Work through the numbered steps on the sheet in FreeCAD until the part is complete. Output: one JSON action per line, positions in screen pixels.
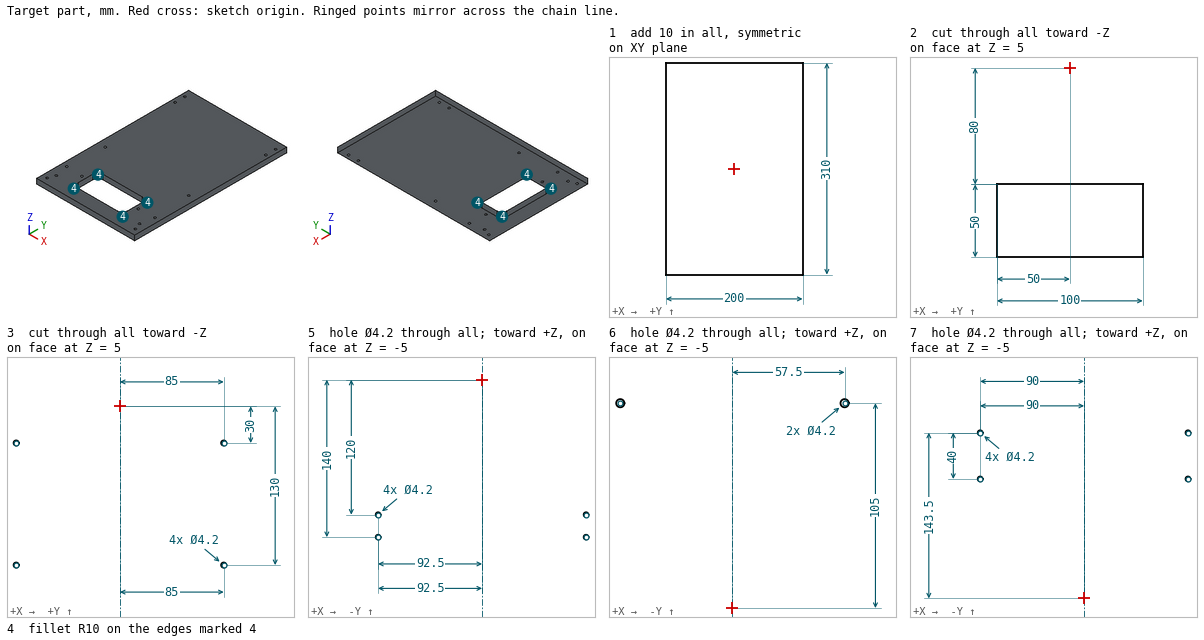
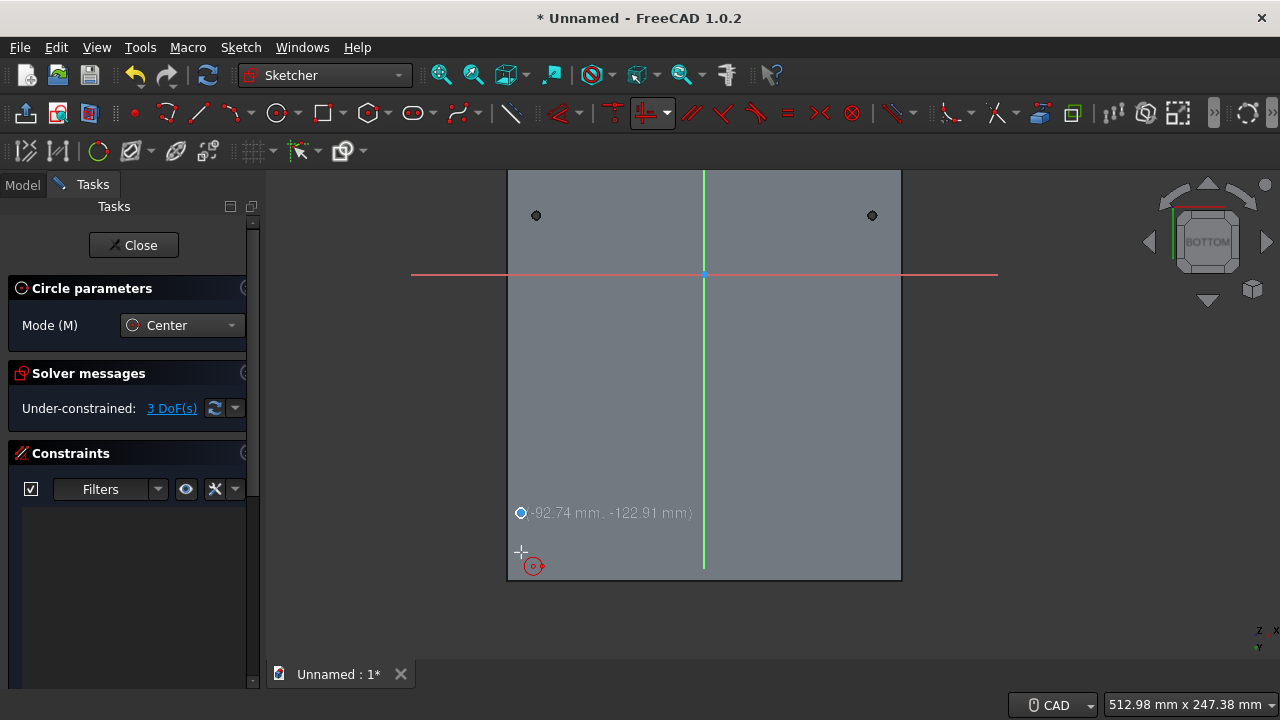
{"action": "left_click", "coordinate": [521, 552]}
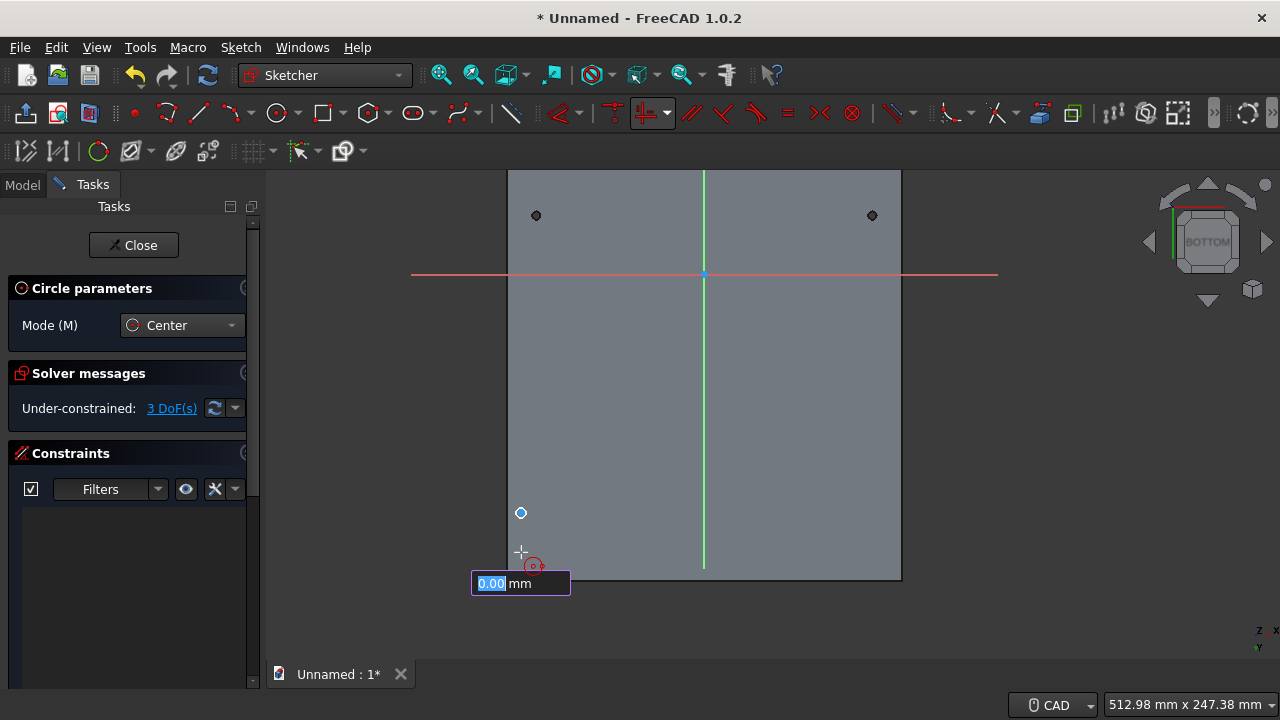
{"action": "scroll", "coordinate": [524, 549], "scroll_direction": "up", "scroll_amount": 7}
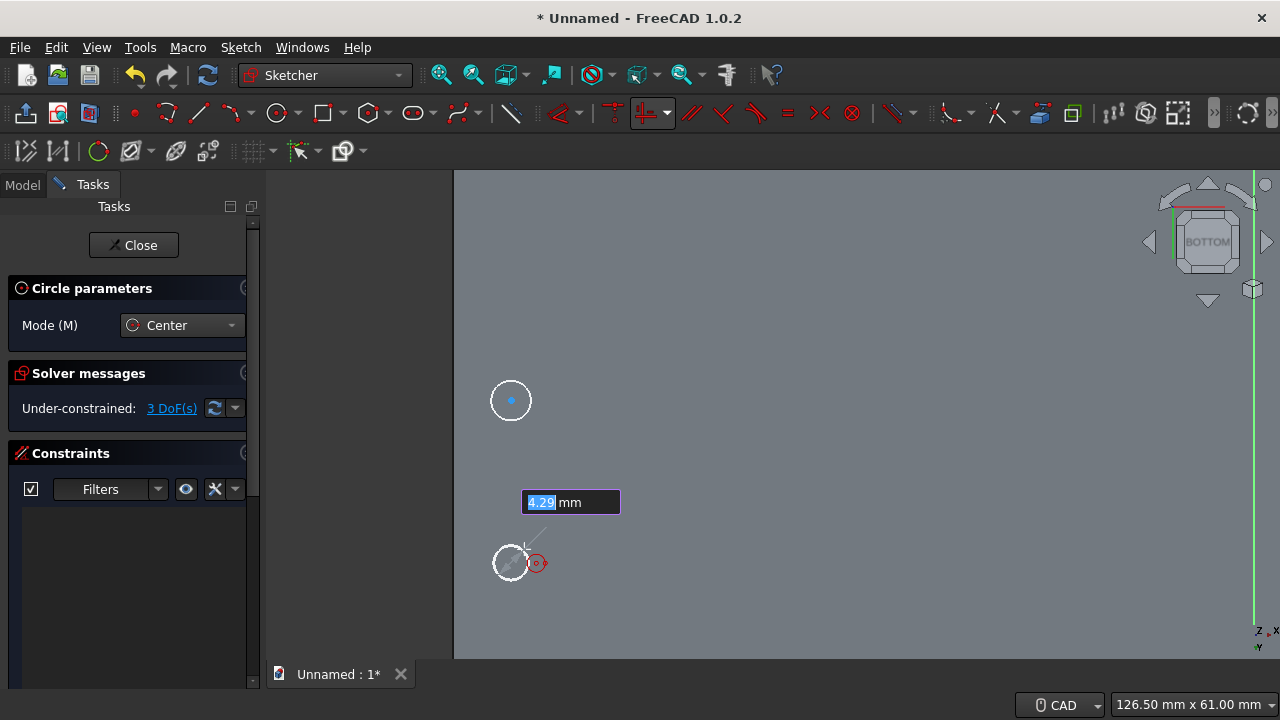
{"action": "left_click", "coordinate": [525, 546]}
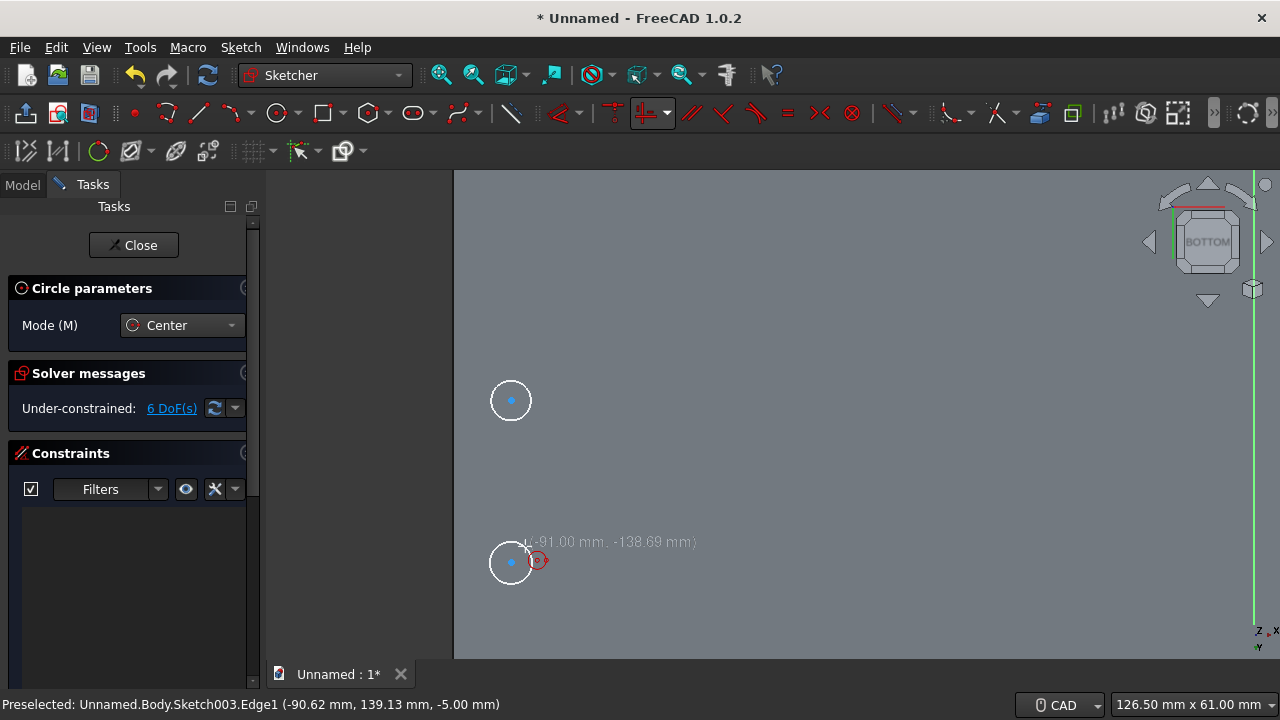
{"action": "scroll", "coordinate": [524, 549], "scroll_direction": "down", "scroll_amount": 7}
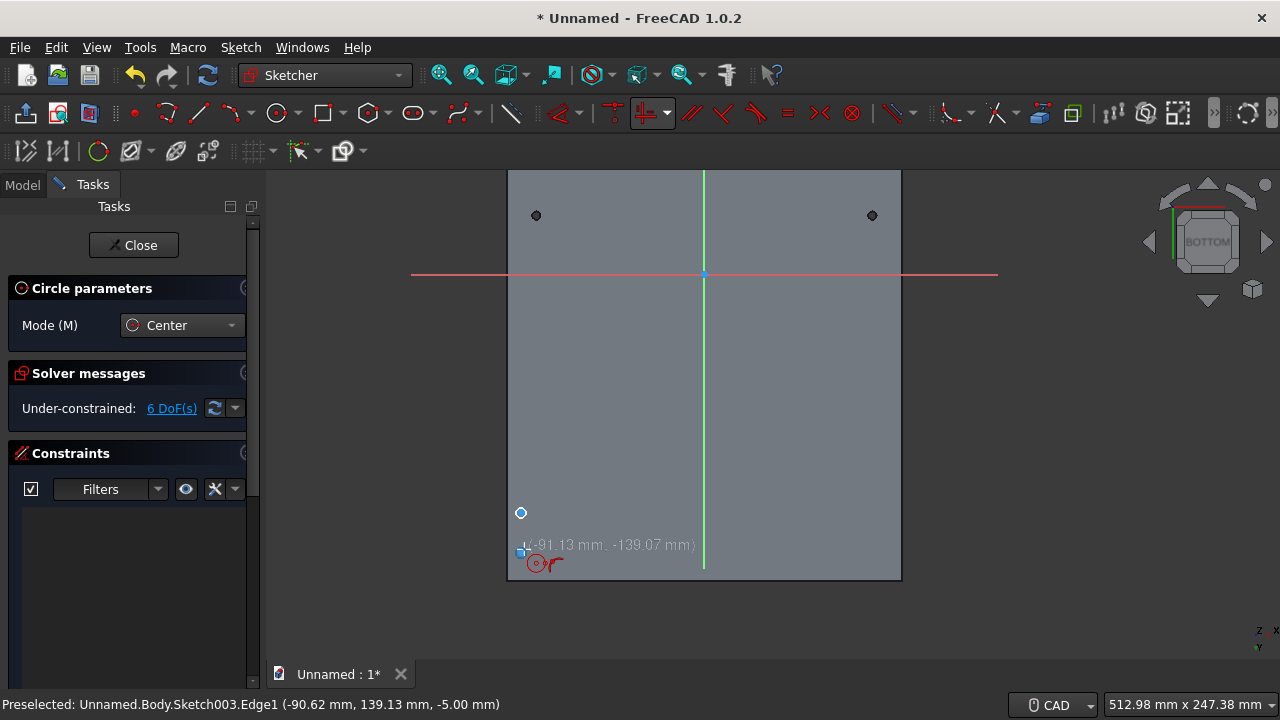
{"action": "scroll", "coordinate": [887, 552], "scroll_direction": "up", "scroll_amount": 9}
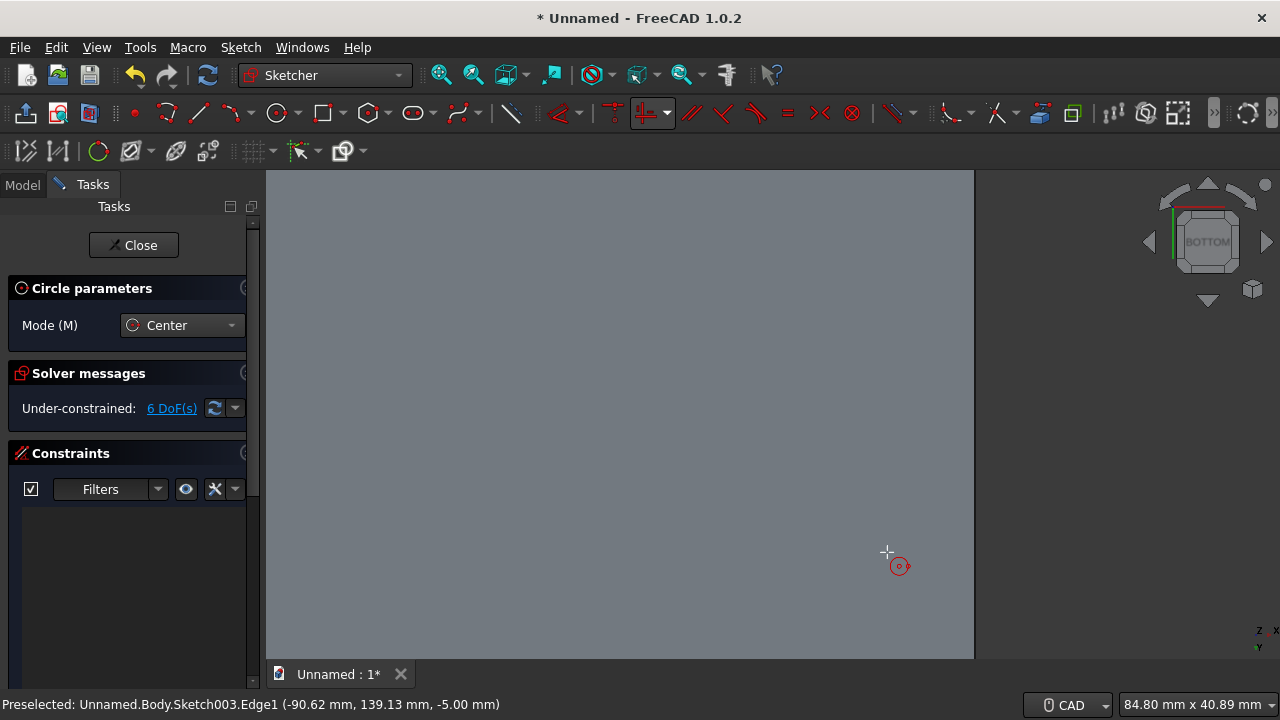
{"action": "scroll", "coordinate": [888, 552], "scroll_direction": "down", "scroll_amount": 9}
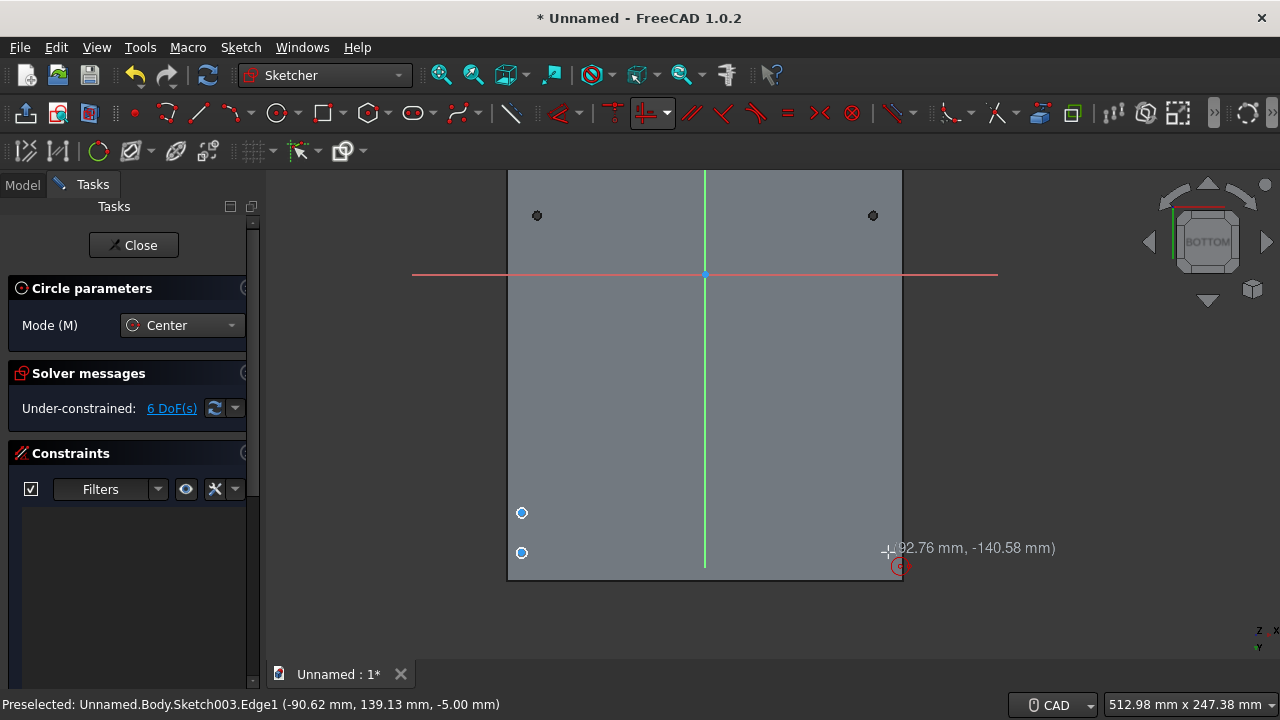
{"action": "left_click", "coordinate": [888, 552]}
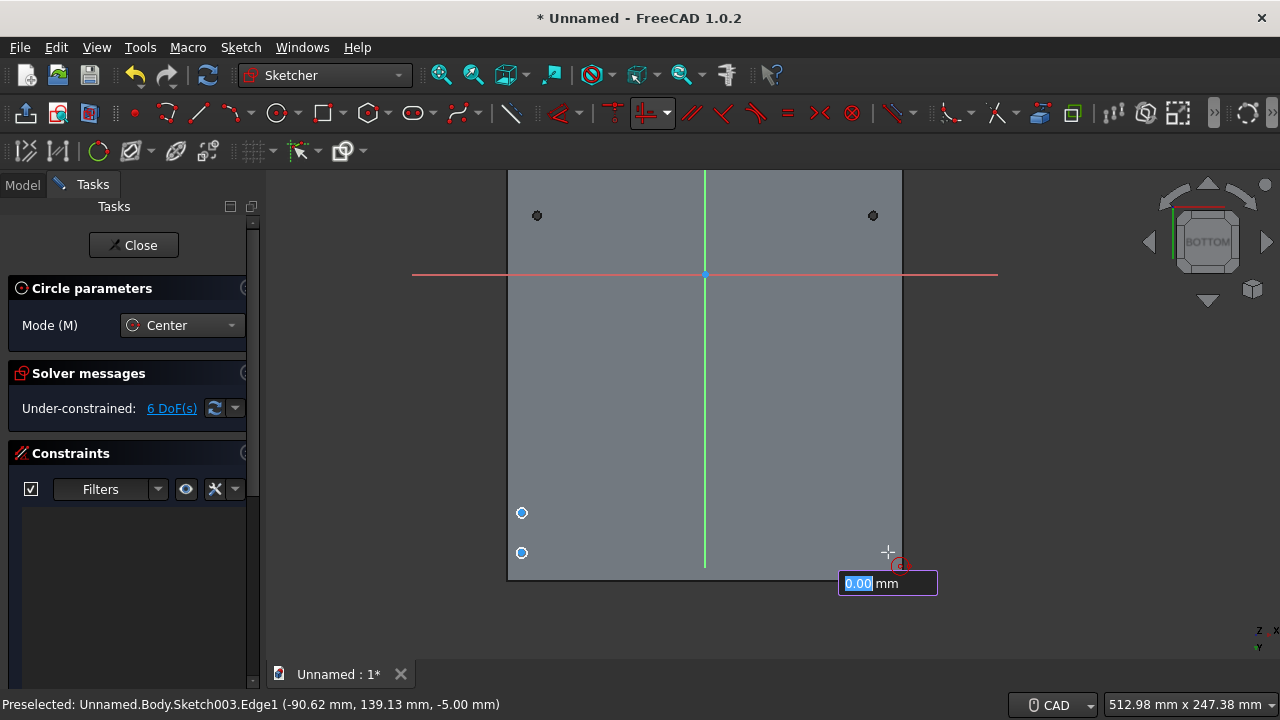
{"action": "scroll", "coordinate": [891, 549], "scroll_direction": "up", "scroll_amount": 7}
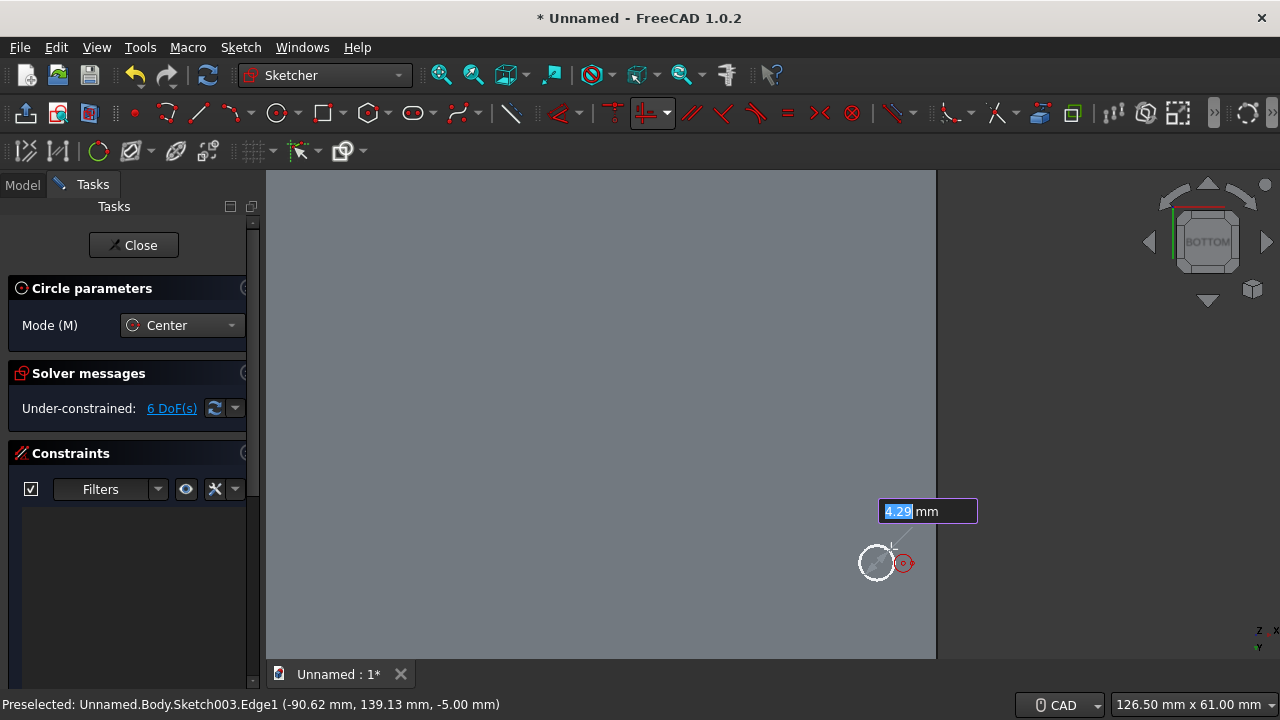
{"action": "left_click", "coordinate": [889, 546]}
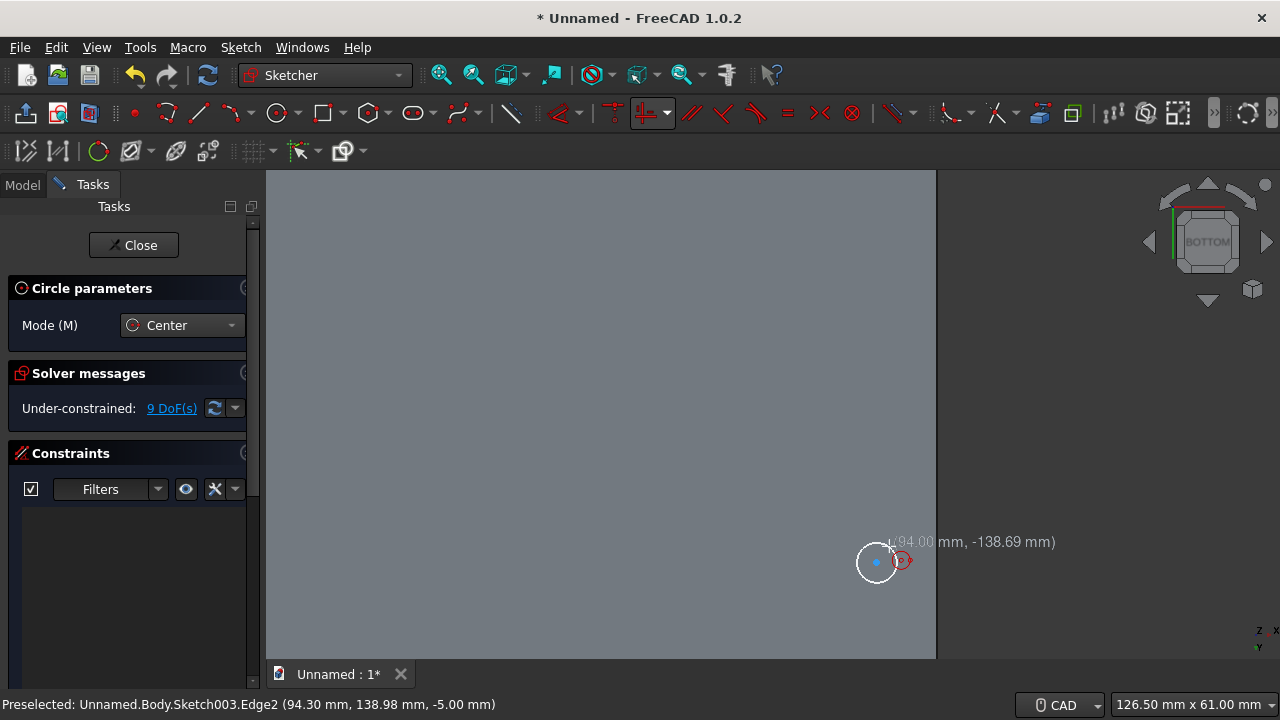
{"action": "scroll", "coordinate": [877, 397], "scroll_direction": "up", "scroll_amount": 2}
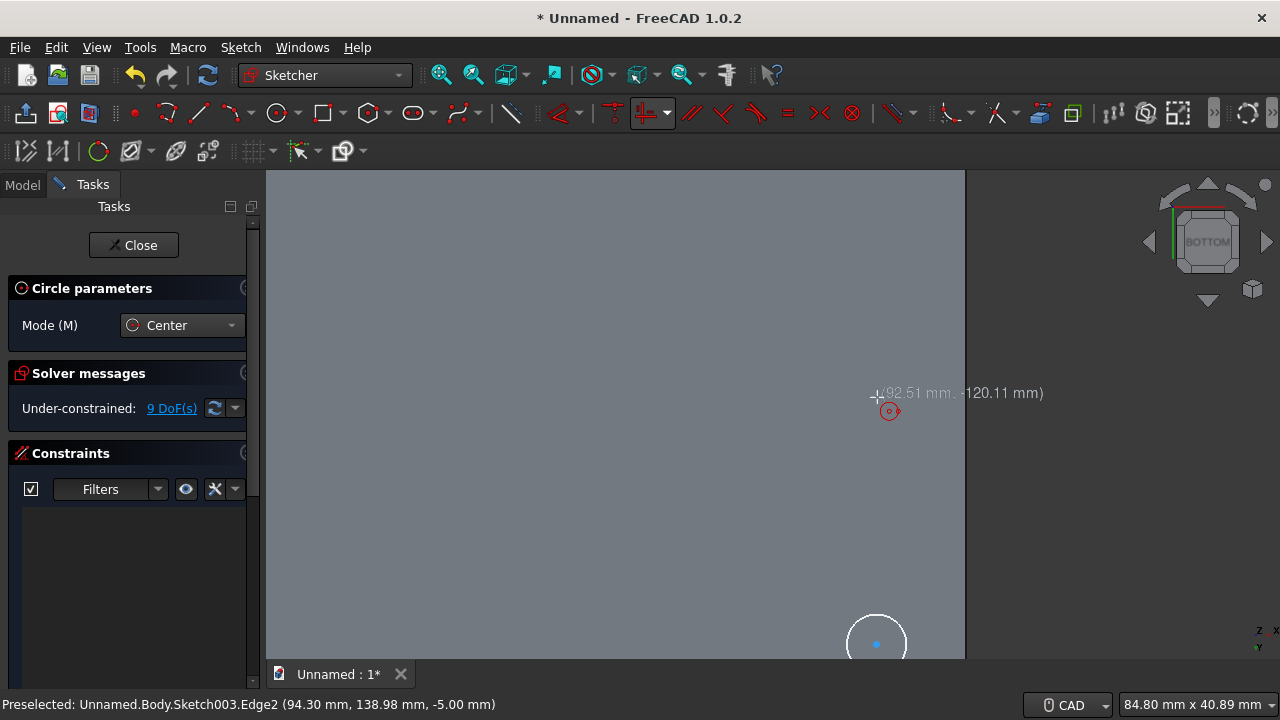
{"action": "scroll", "coordinate": [889, 534], "scroll_direction": "down", "scroll_amount": 9}